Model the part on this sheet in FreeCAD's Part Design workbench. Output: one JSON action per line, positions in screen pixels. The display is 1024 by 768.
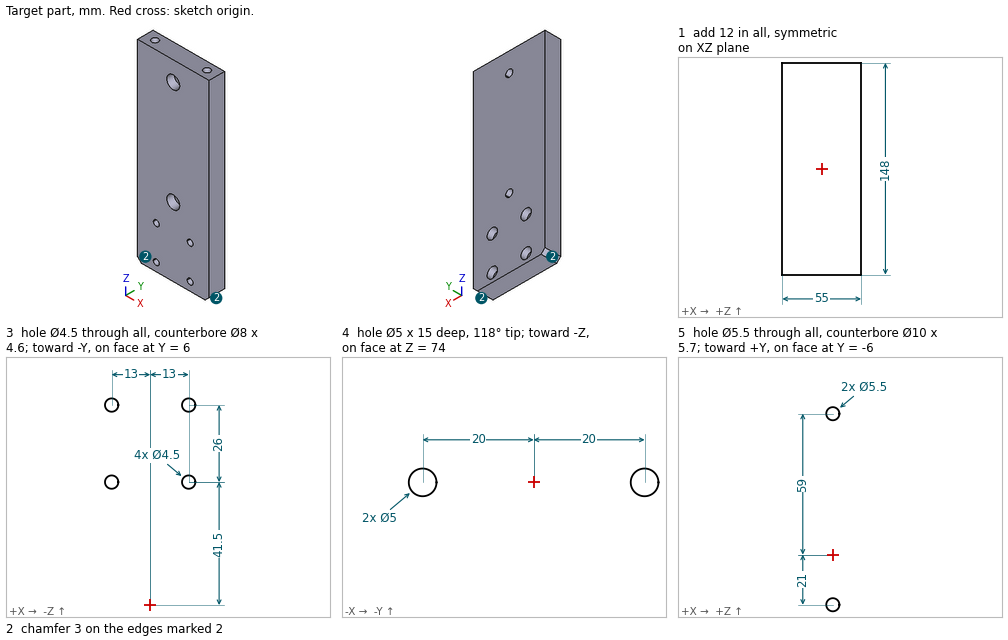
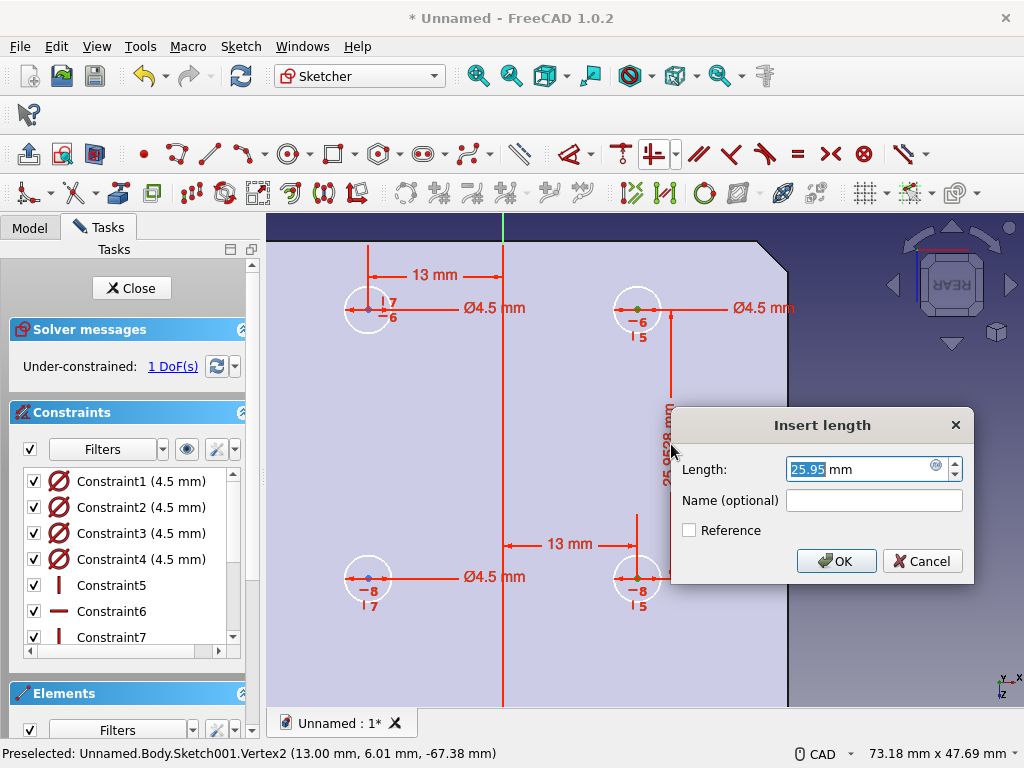
{"action": "type", "text": "26"}
{"action": "key", "text": "Return"}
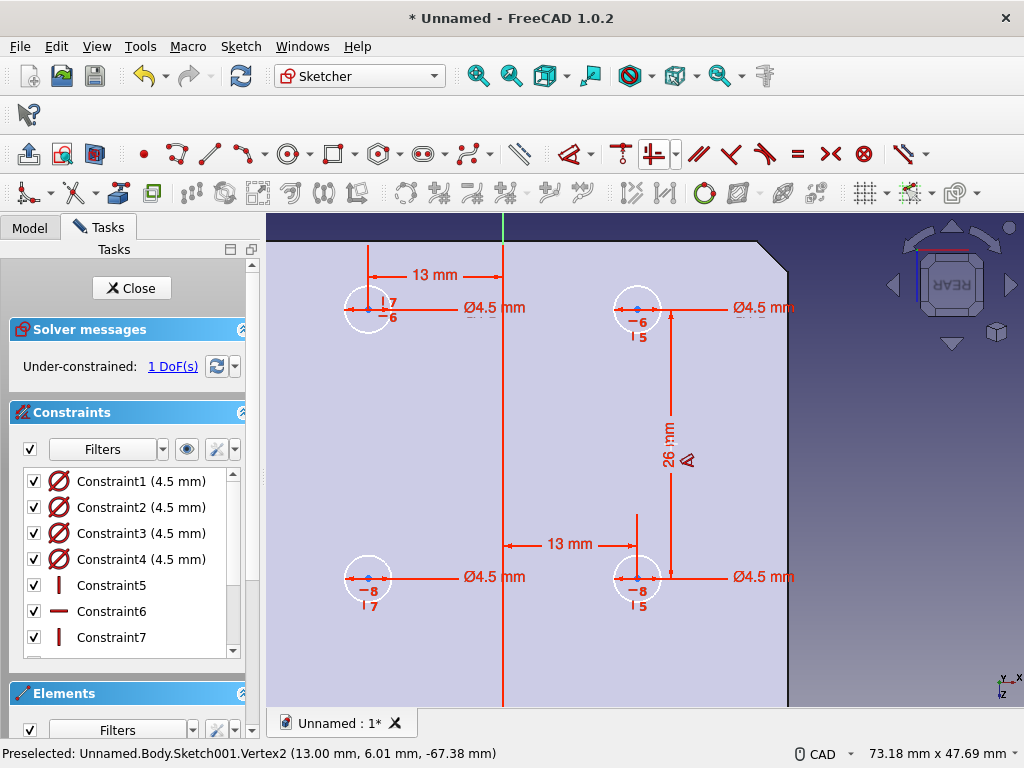
{"action": "left_click", "coordinate": [637, 579]}
{"action": "left_click", "coordinate": [671, 629]}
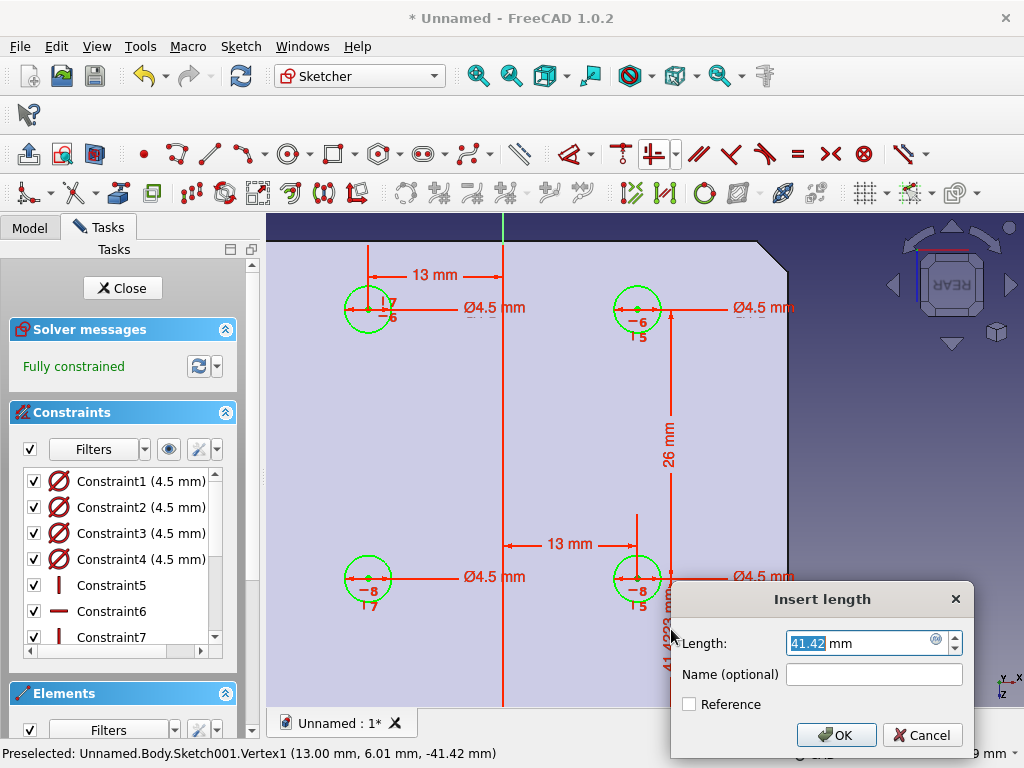
{"action": "type", "text": "41.5"}
{"action": "key", "text": "Return"}
{"action": "key", "text": "Escape"}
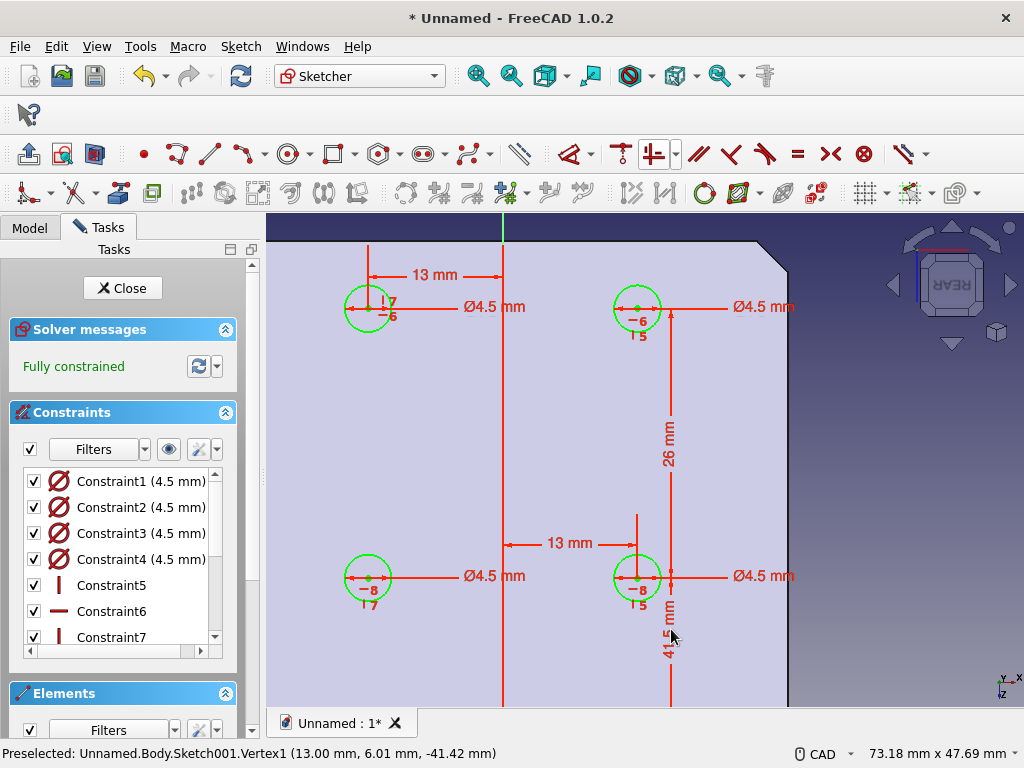
{"action": "left_click", "coordinate": [123, 288]}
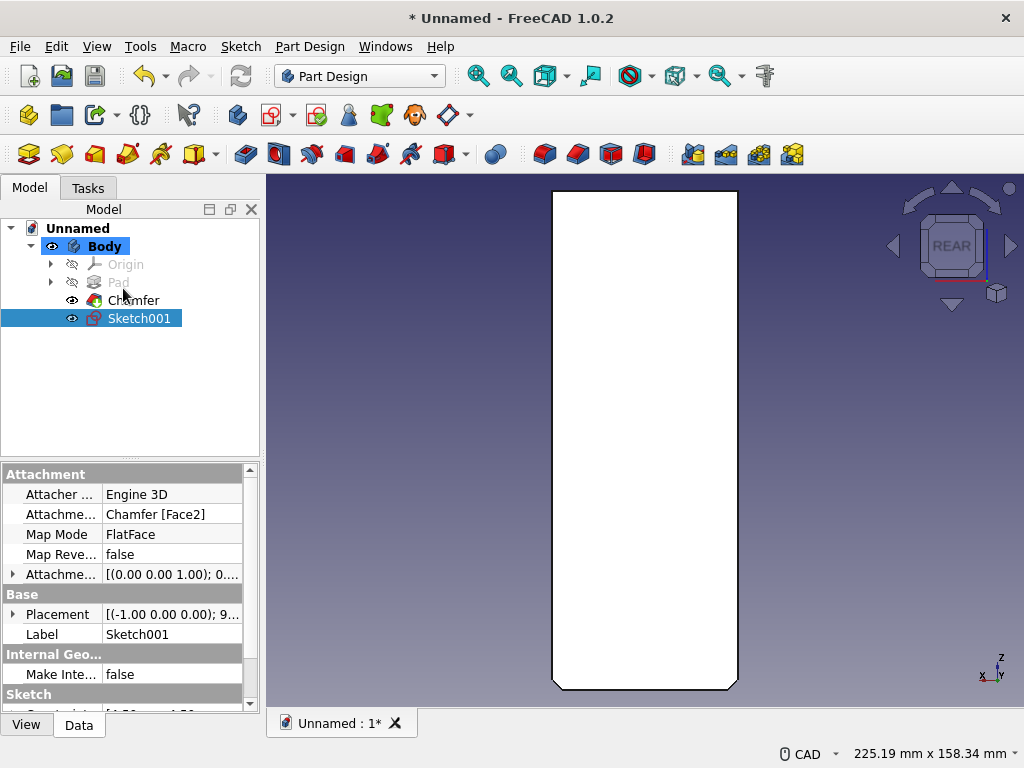
{"action": "left_click", "coordinate": [279, 154]}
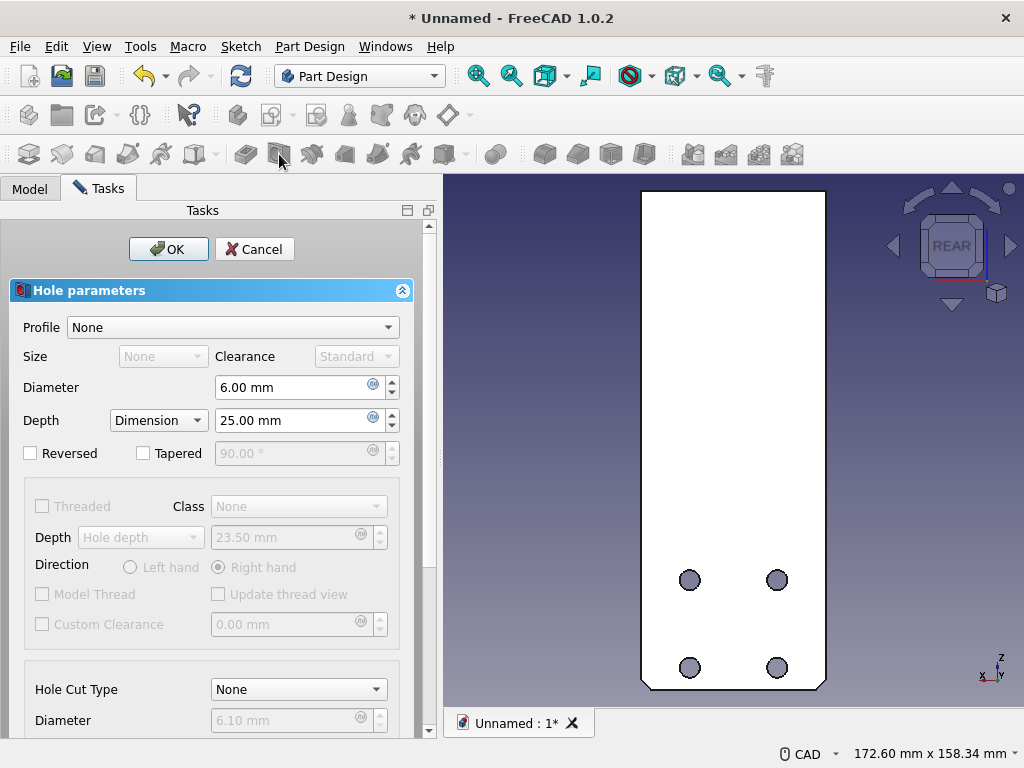
{"action": "triple_click", "coordinate": [300, 388]}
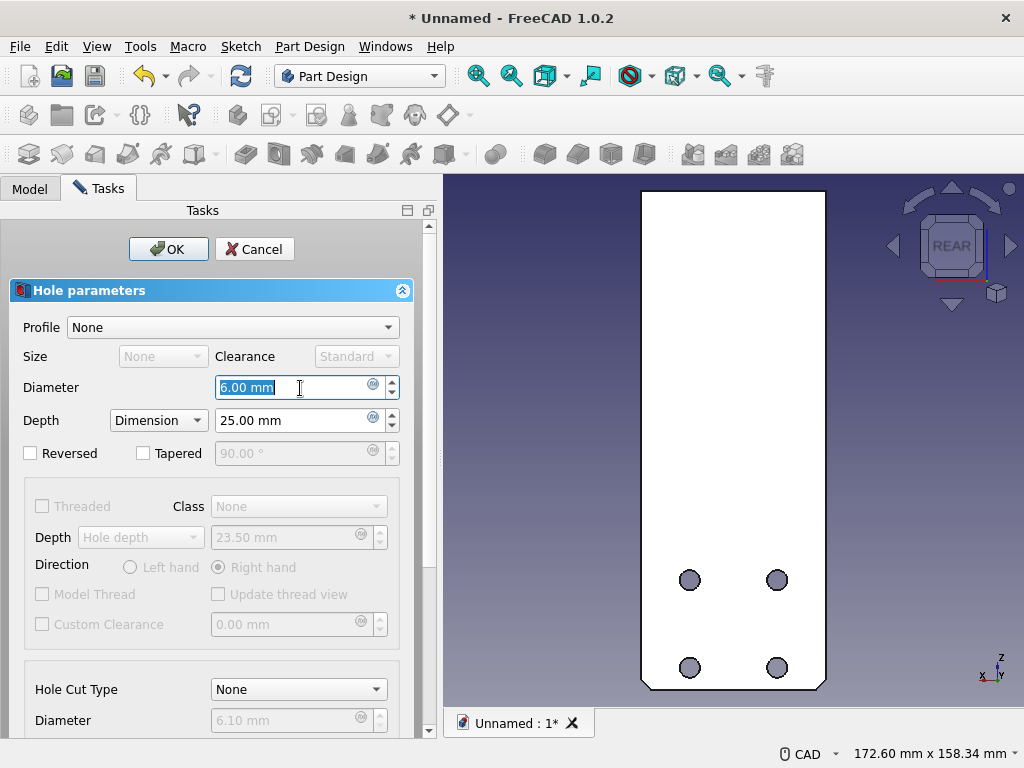
{"action": "type", "text": "4.5"}
{"action": "key", "text": "Tab"}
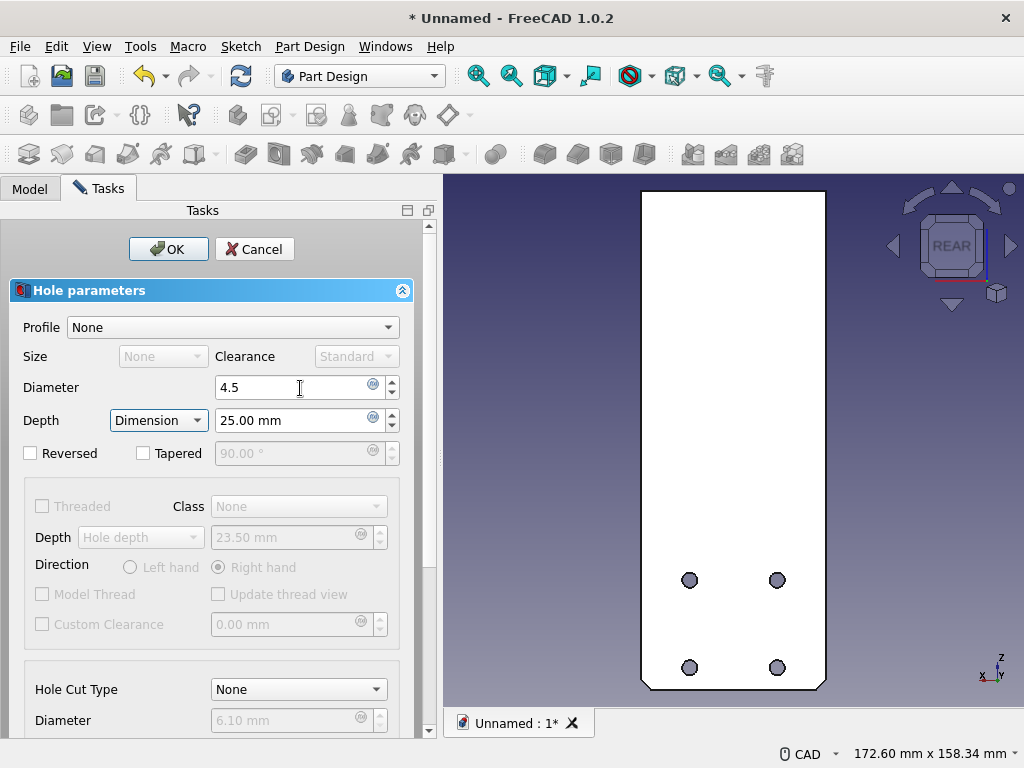
{"action": "left_click", "coordinate": [160, 420]}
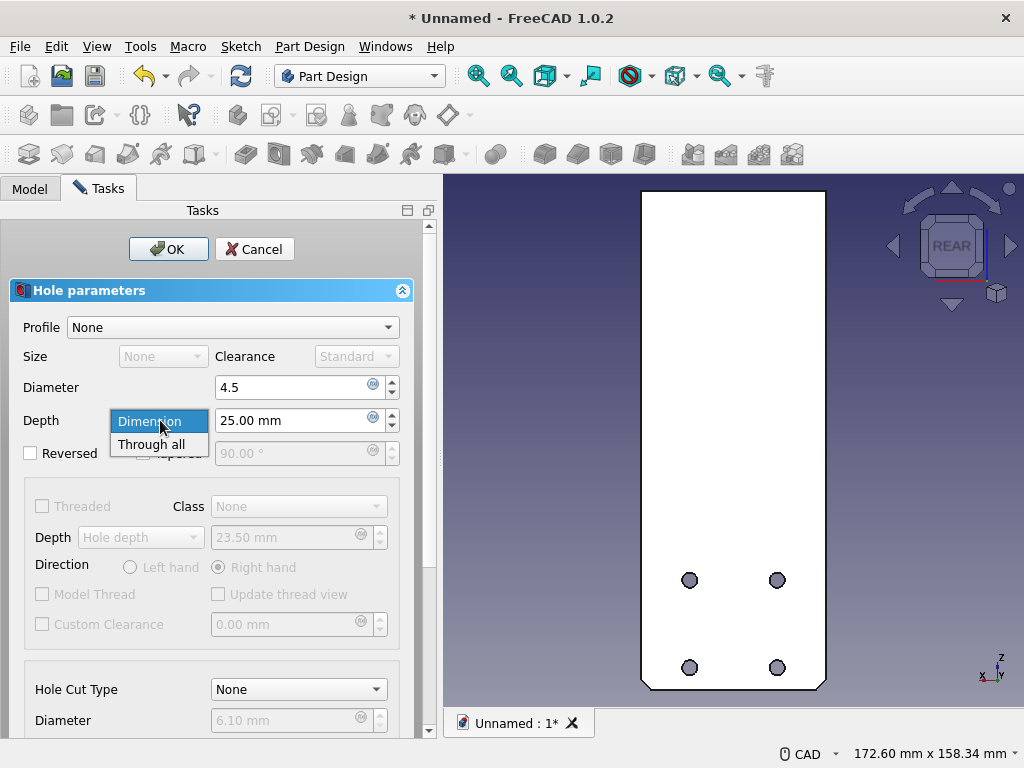
{"action": "left_click", "coordinate": [158, 444]}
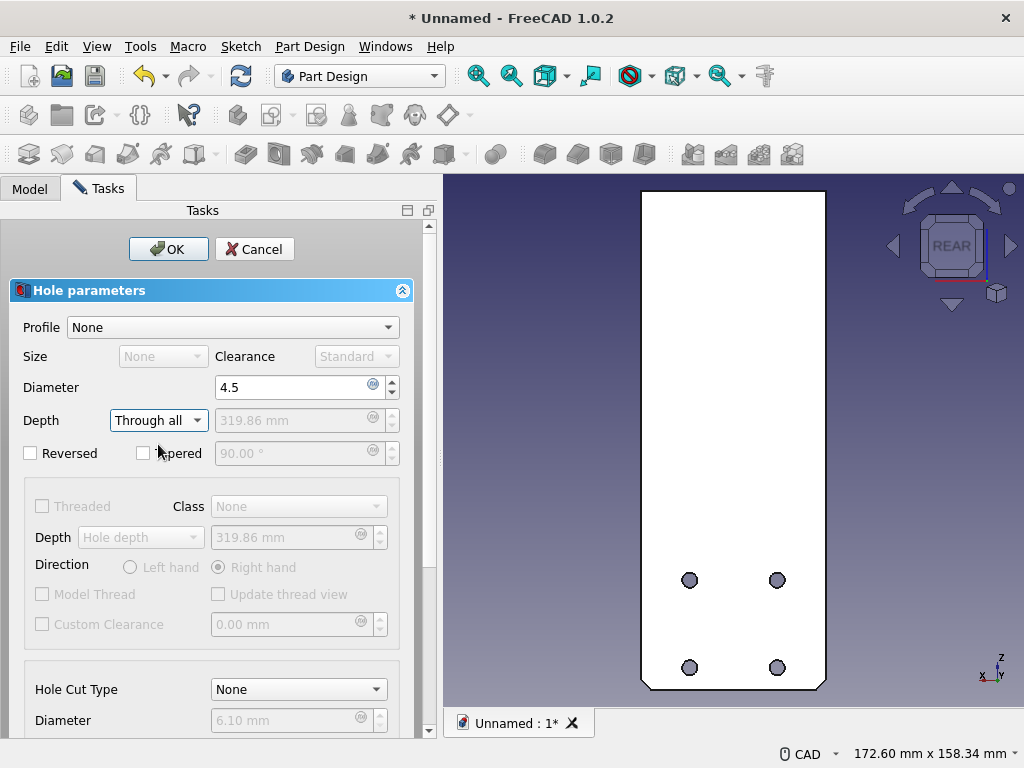
{"action": "left_click", "coordinate": [300, 690]}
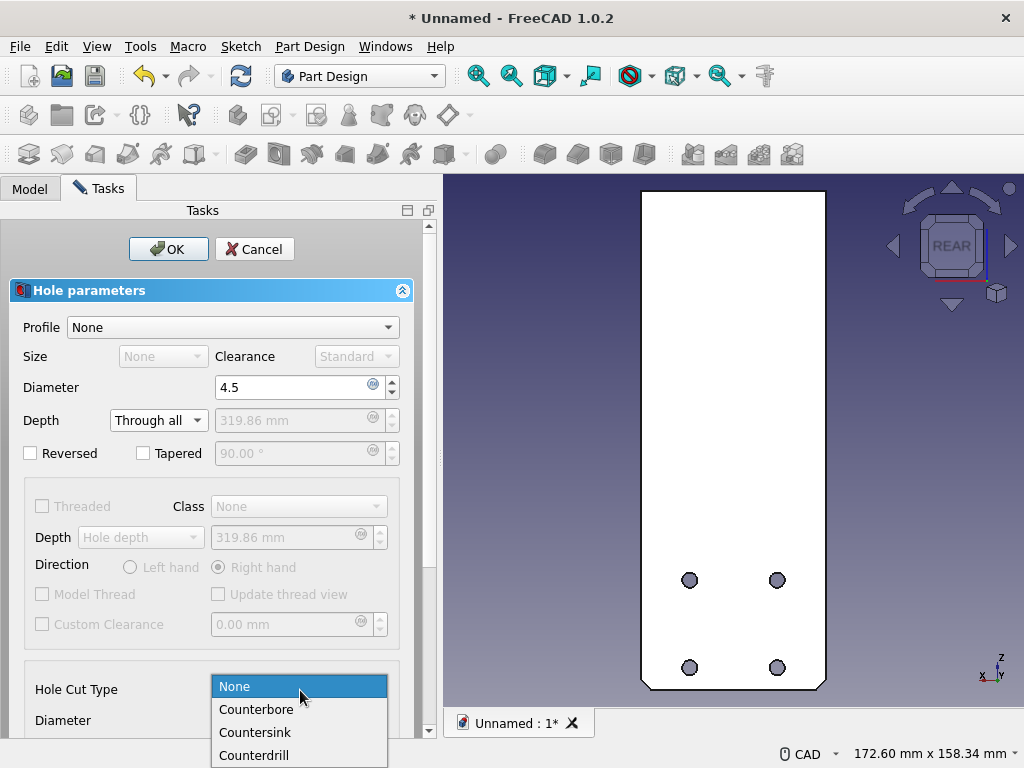
{"action": "left_click", "coordinate": [298, 710]}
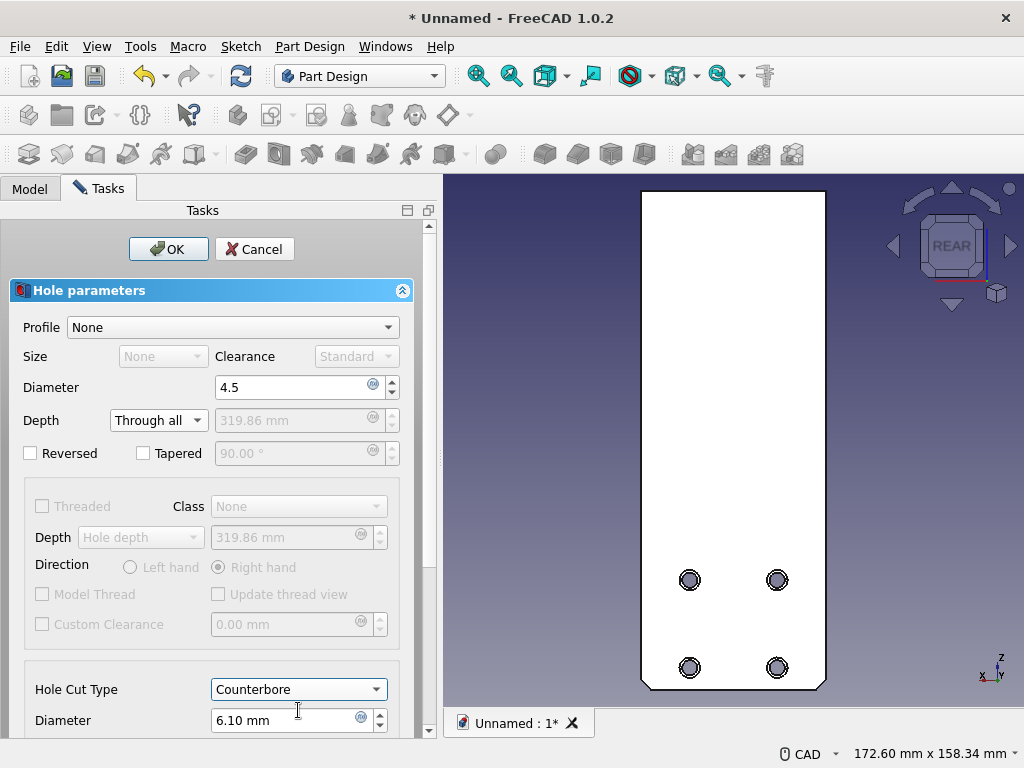
{"action": "triple_click", "coordinate": [292, 720]}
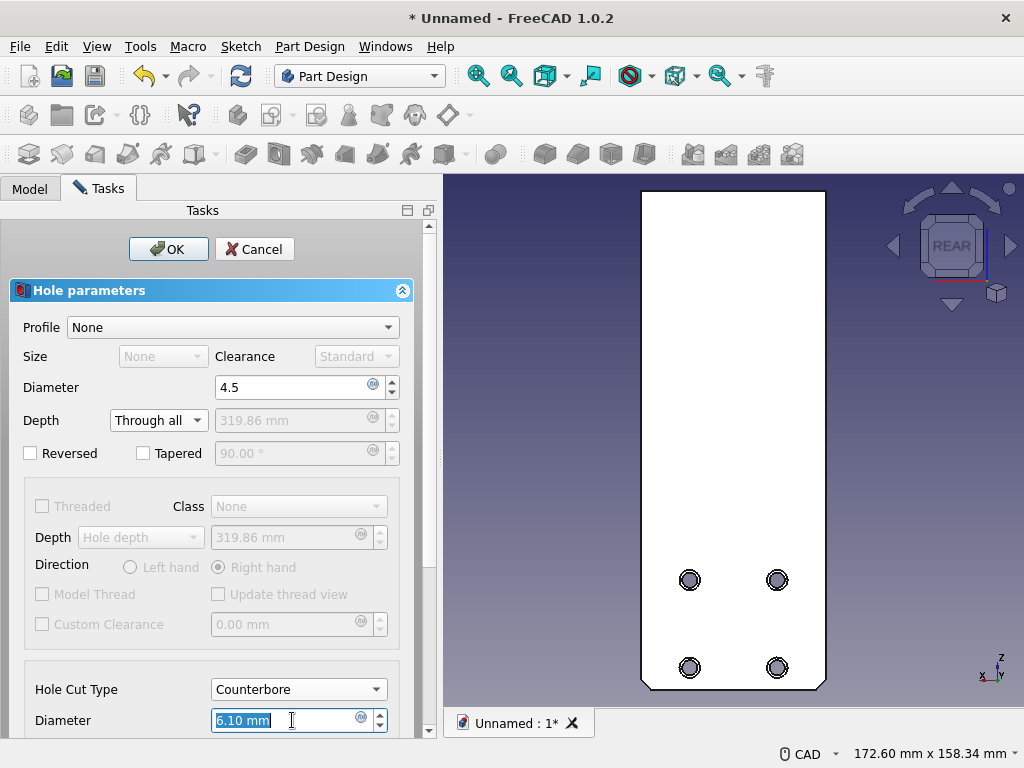
{"action": "type", "text": "8"}
{"action": "key", "text": "Tab"}